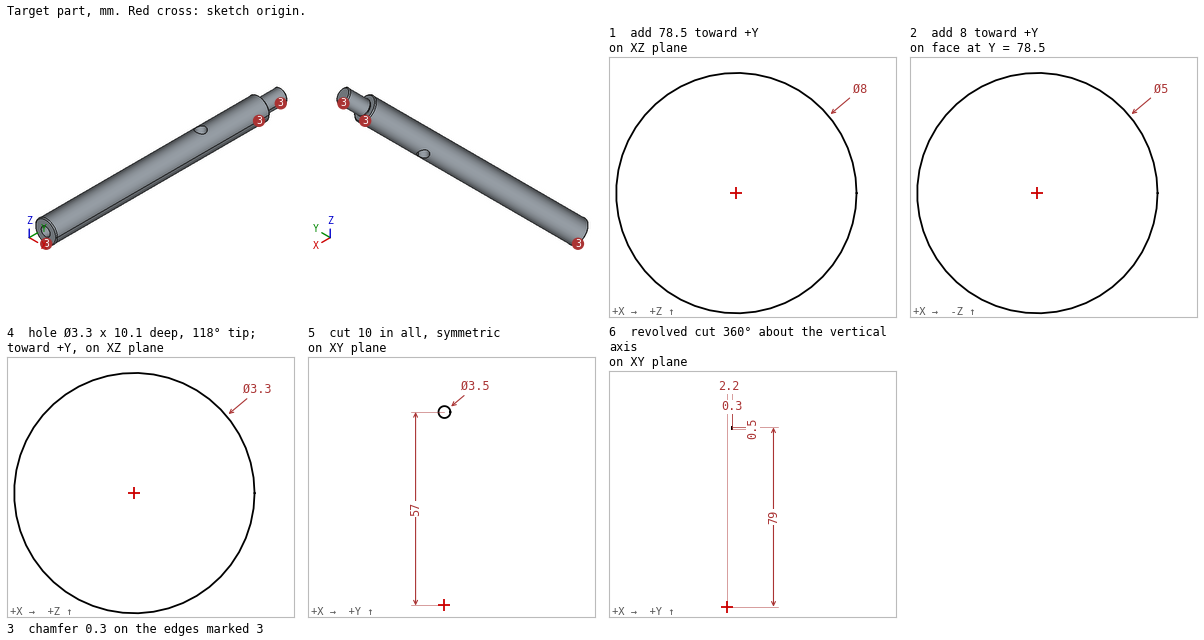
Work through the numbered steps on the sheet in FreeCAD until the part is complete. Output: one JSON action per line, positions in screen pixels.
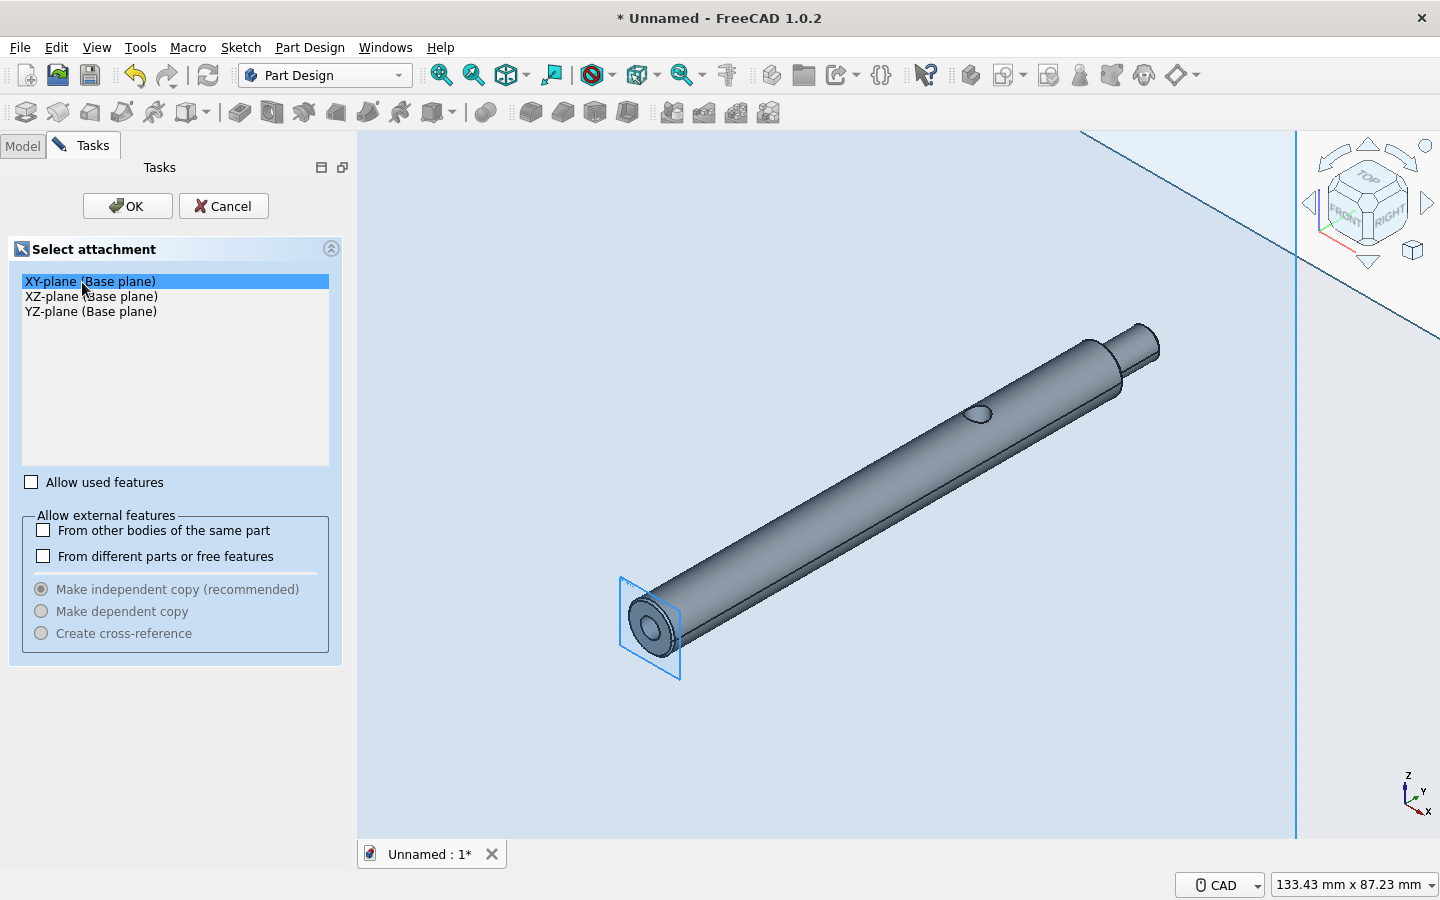
{"action": "left_click", "coordinate": [128, 206]}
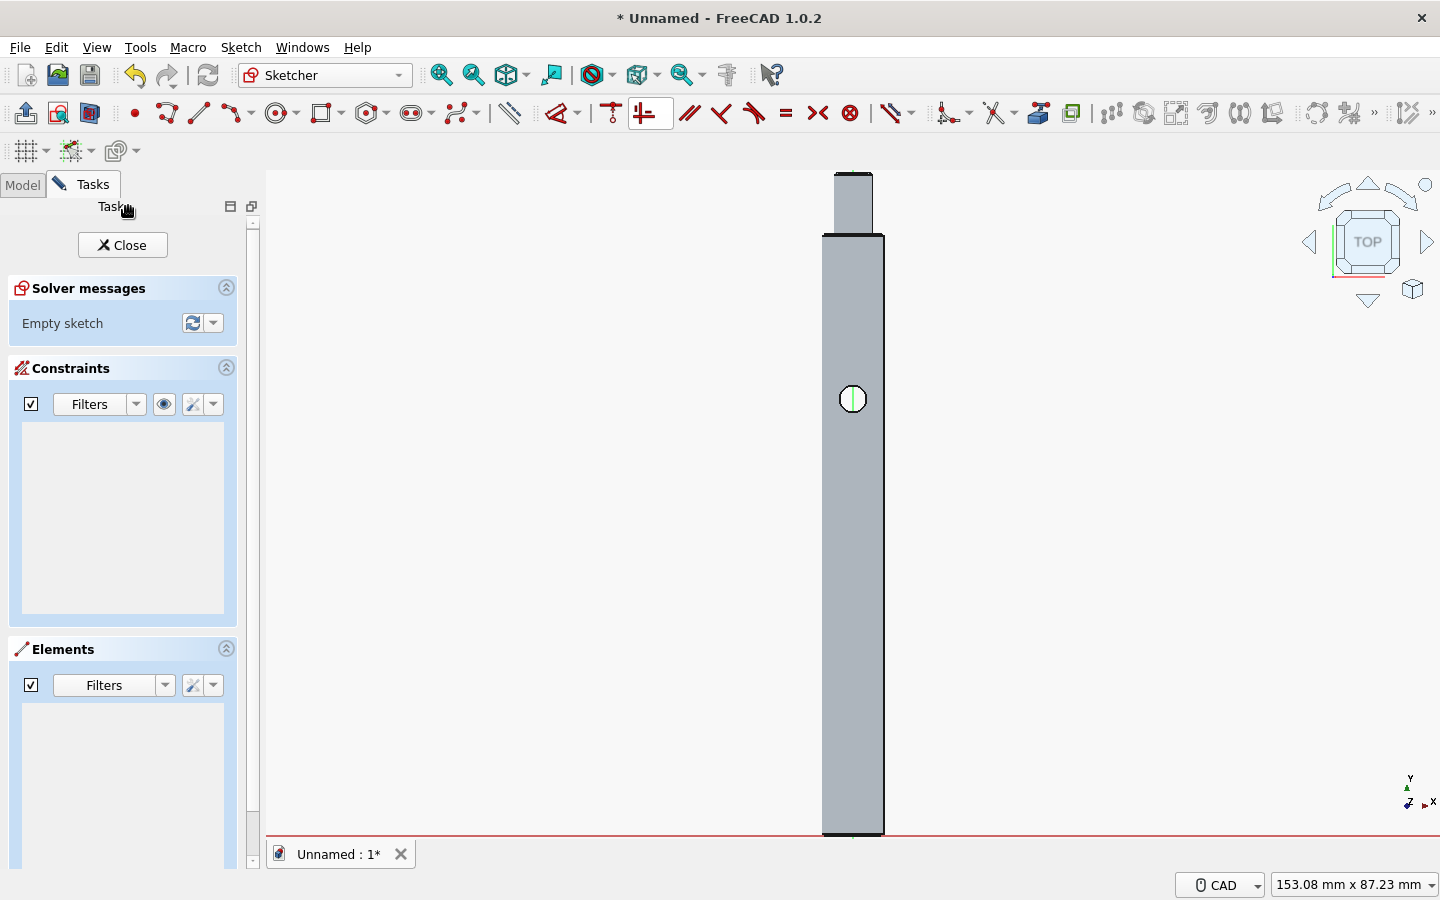
{"action": "key", "text": "q s"}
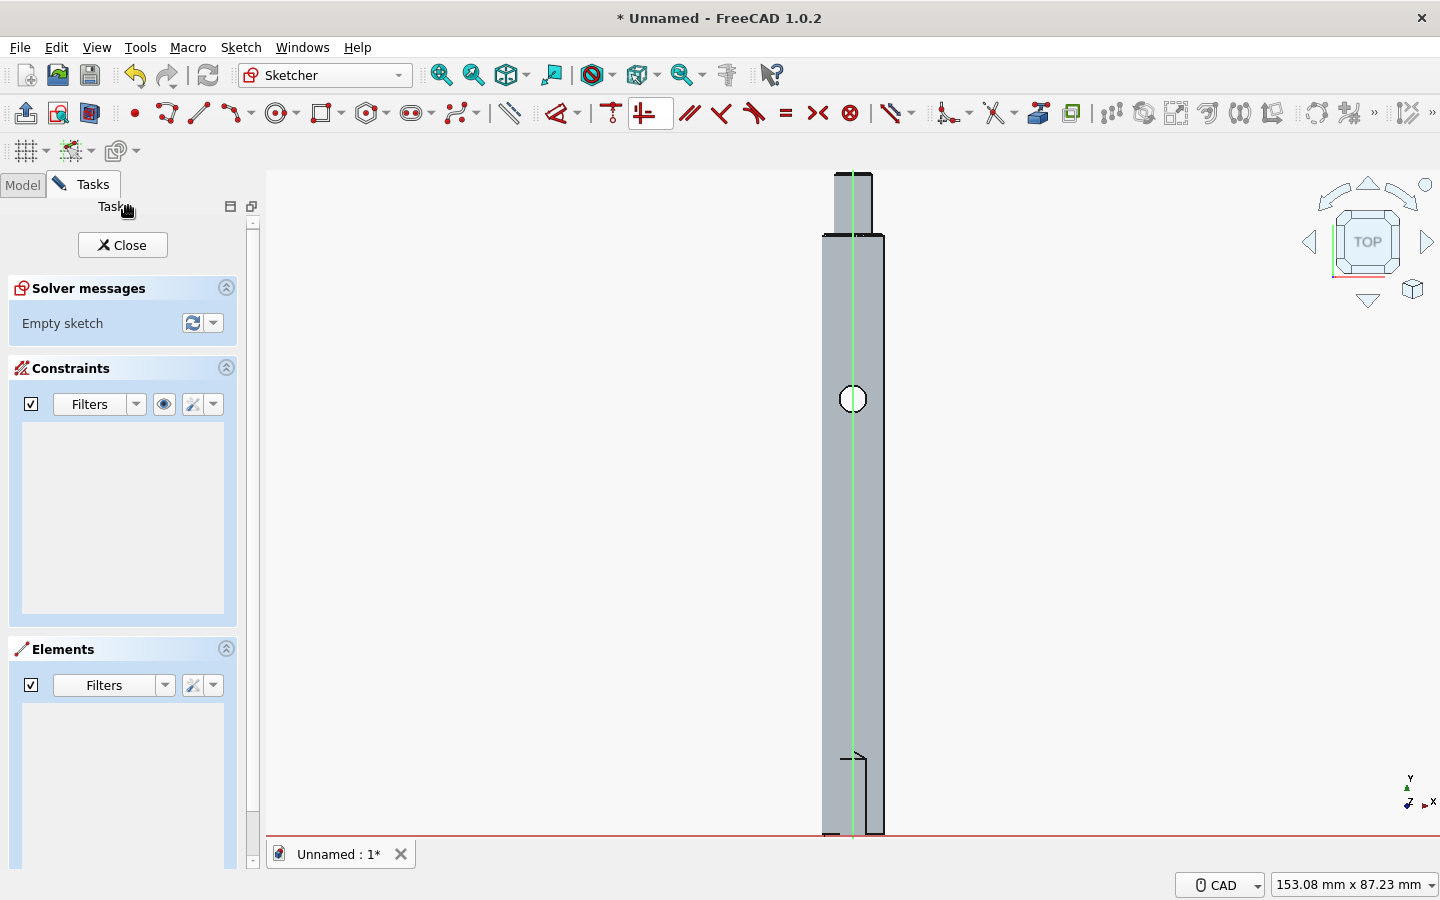
{"action": "scroll", "coordinate": [876, 218], "scroll_direction": "up", "scroll_amount": 15}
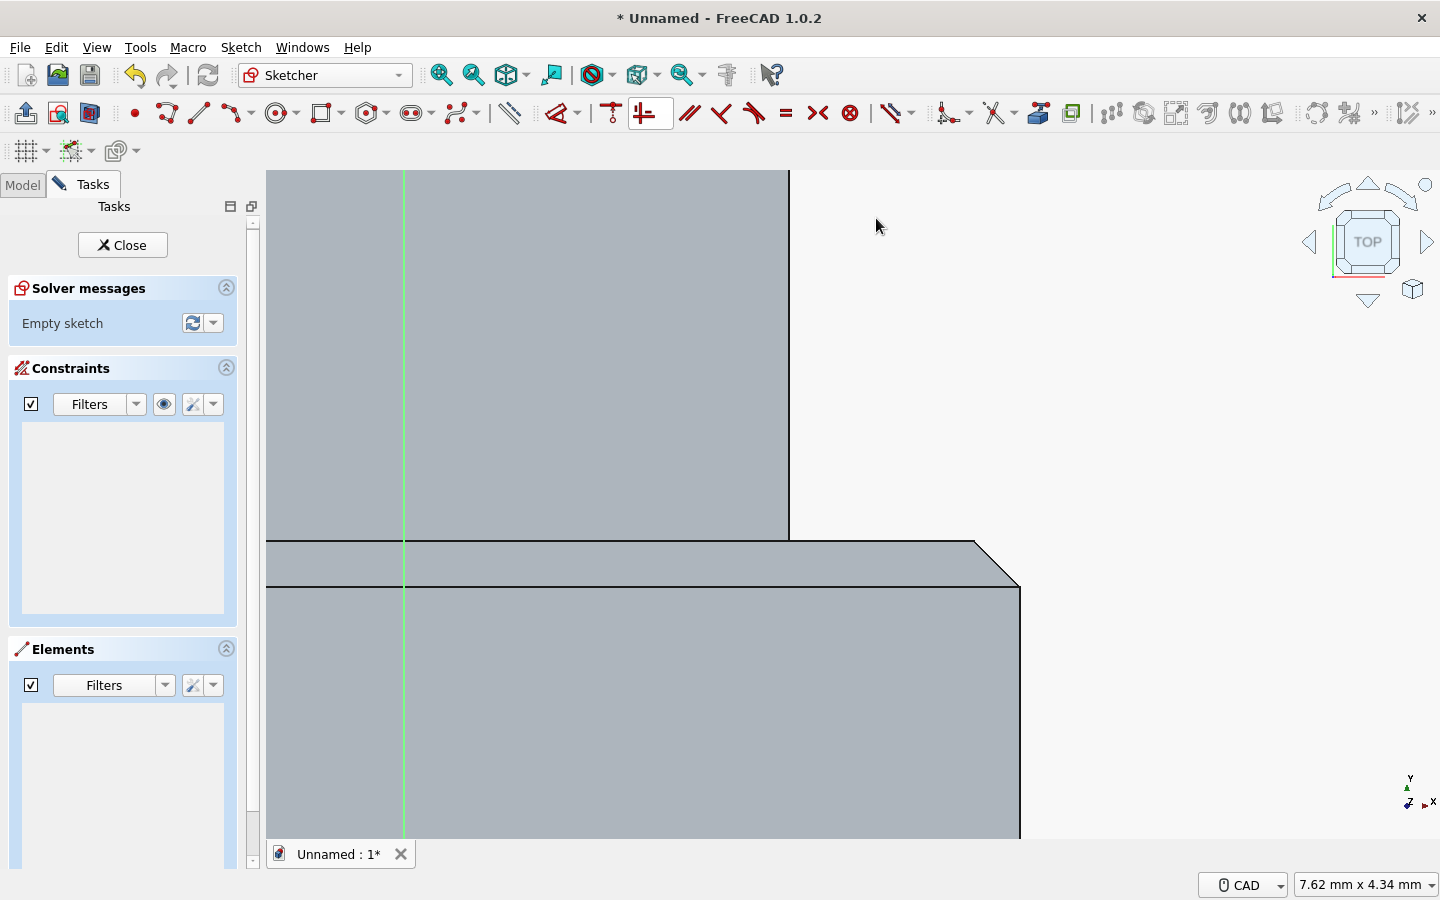
{"action": "scroll", "coordinate": [762, 502], "scroll_direction": "up", "scroll_amount": 9}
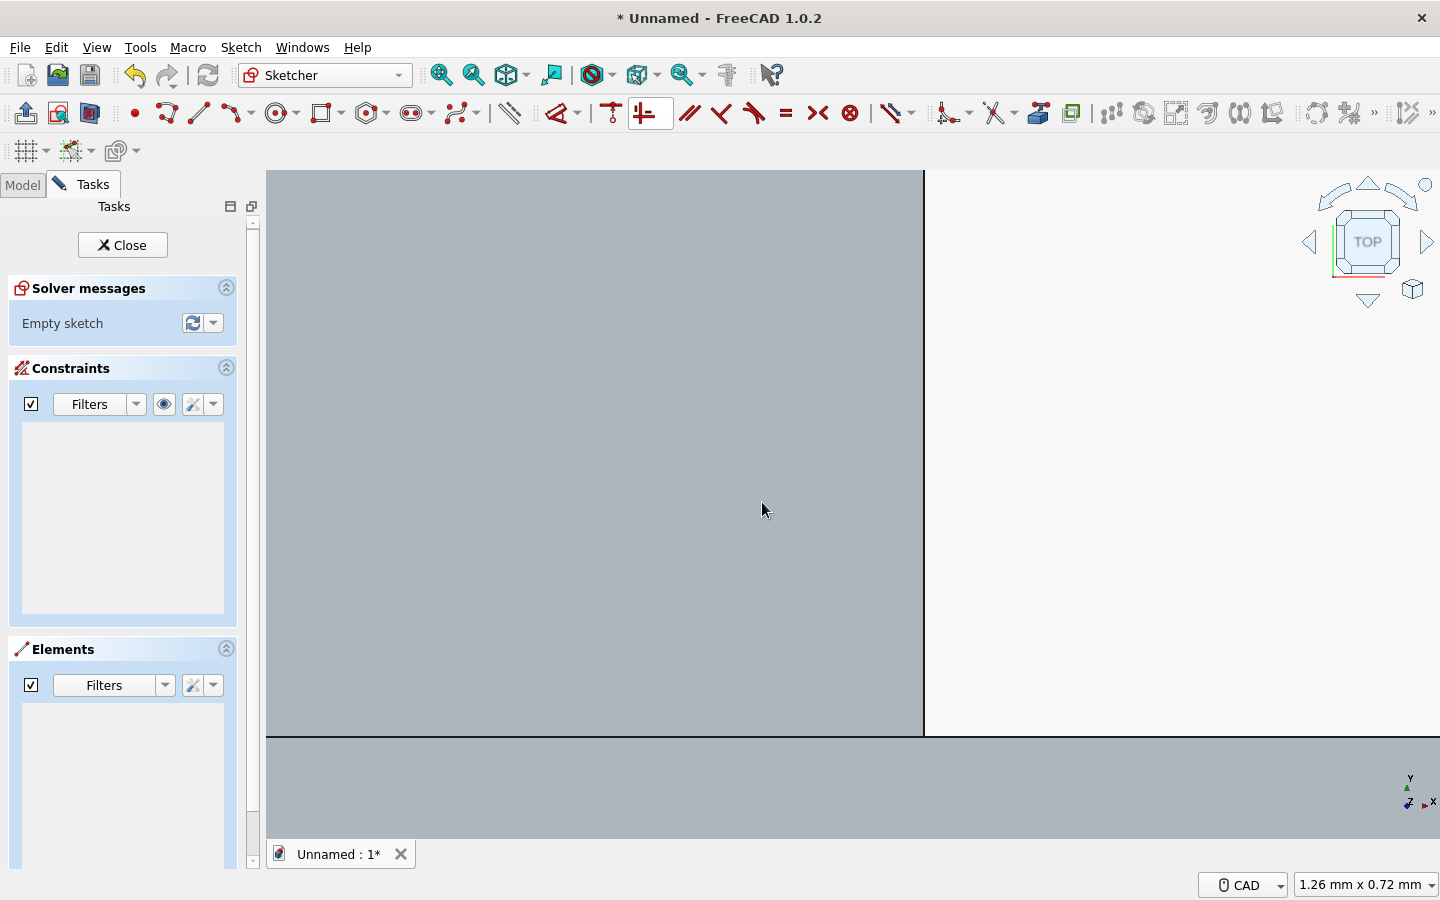
{"action": "left_click", "coordinate": [322, 114]}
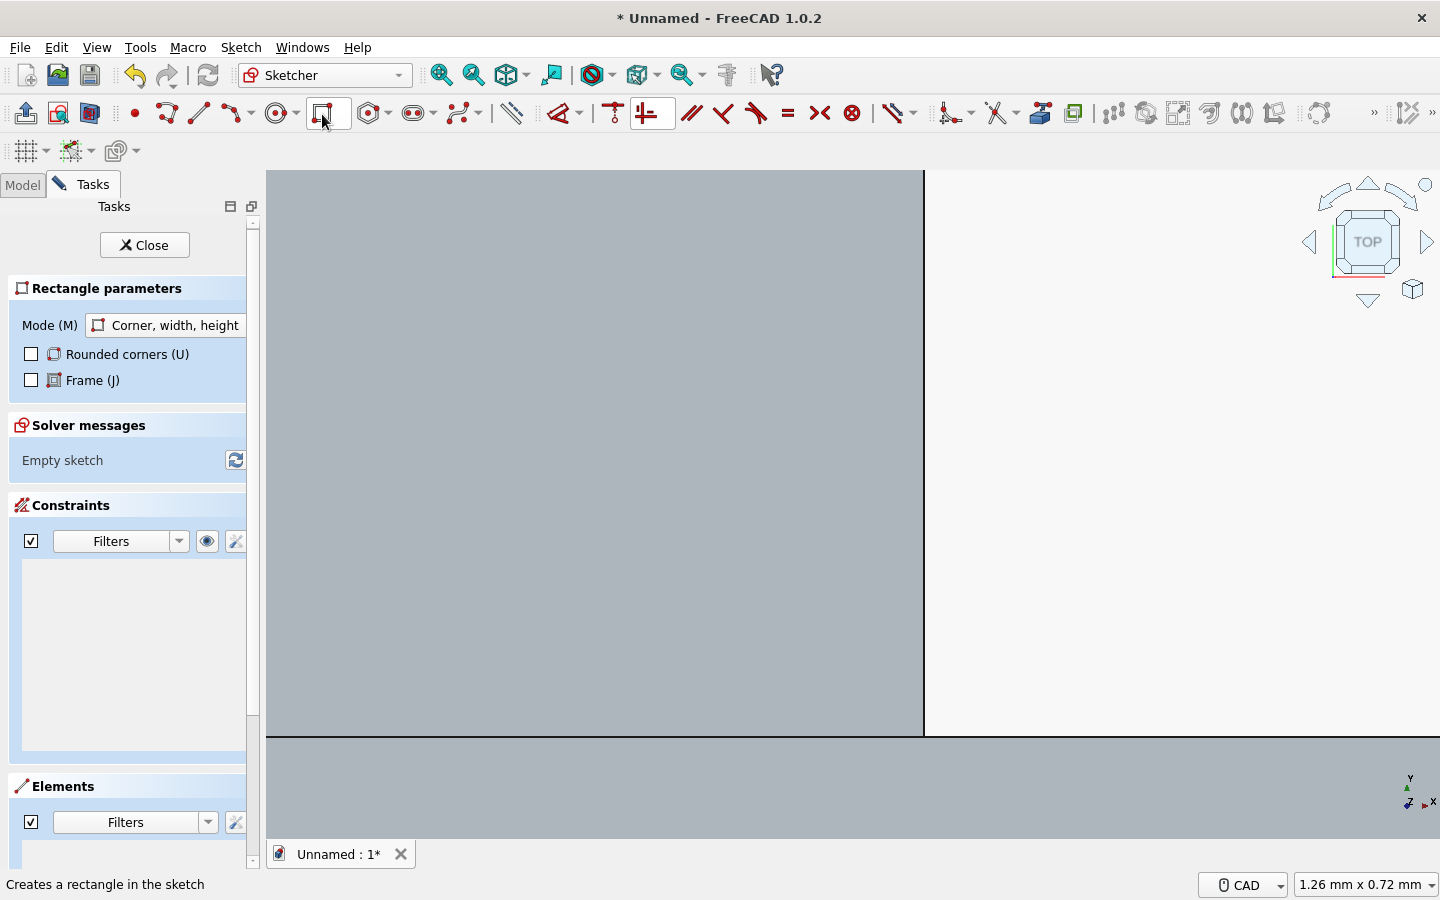
{"action": "left_click", "coordinate": [645, 271]}
{"action": "left_click", "coordinate": [924, 737]}
{"action": "key", "text": "Escape"}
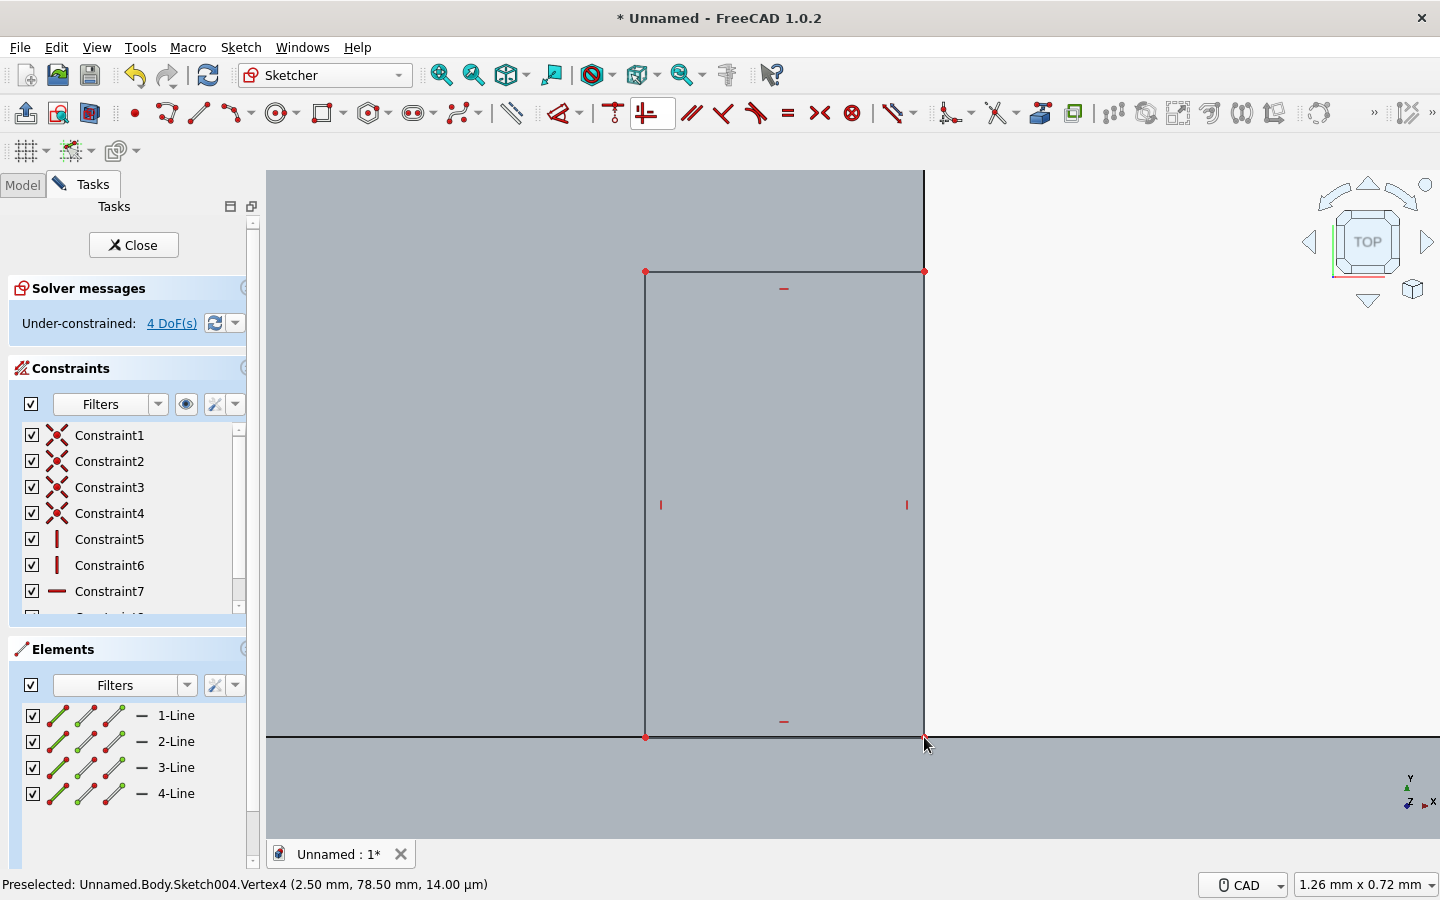
{"action": "key", "text": "d"}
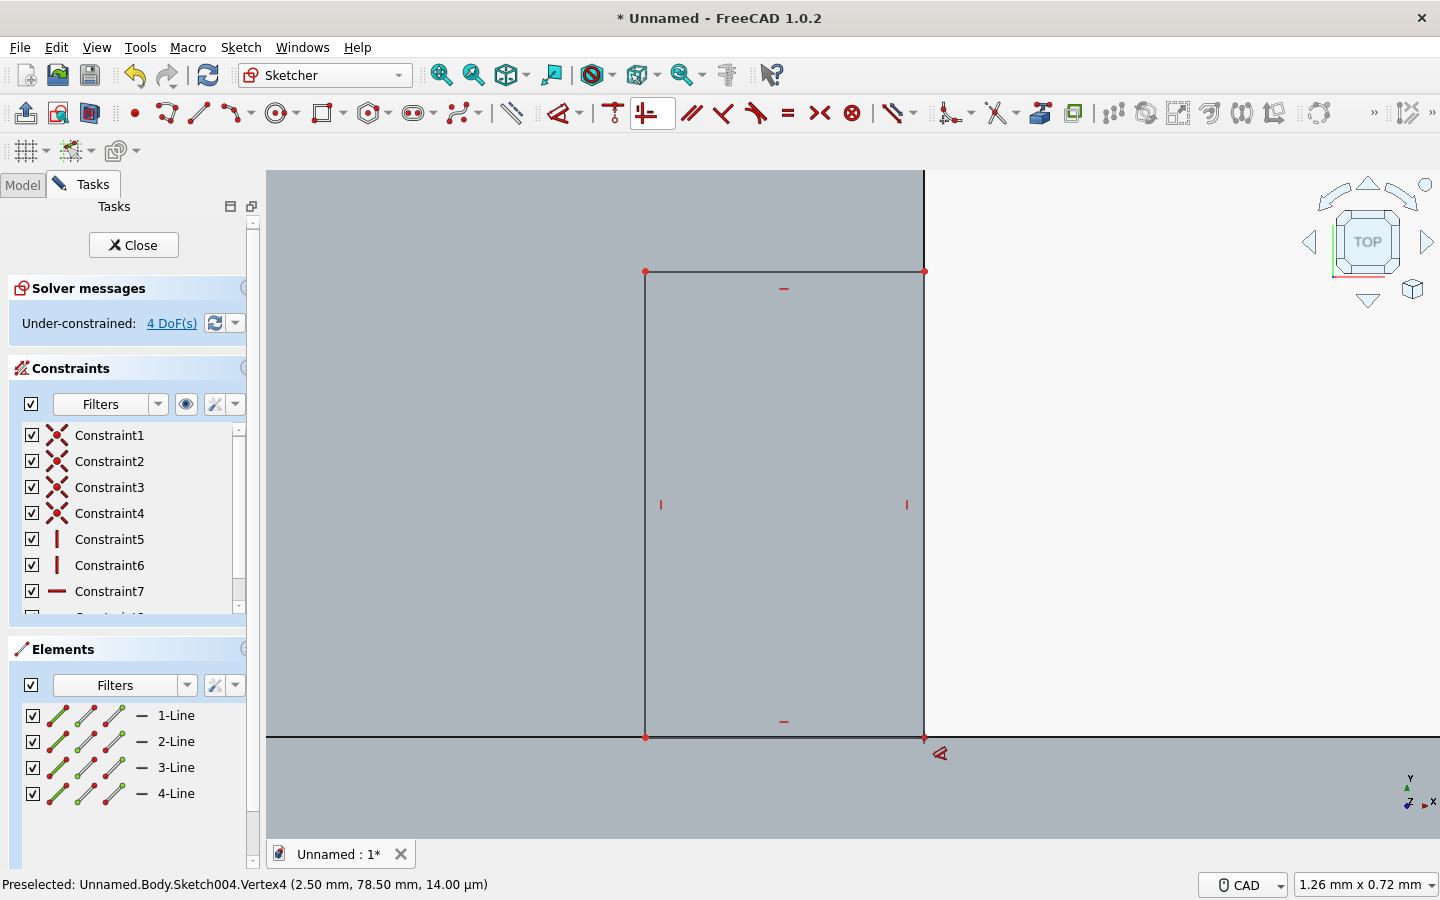
{"action": "left_click", "coordinate": [645, 412]}
{"action": "left_click", "coordinate": [611, 505]}